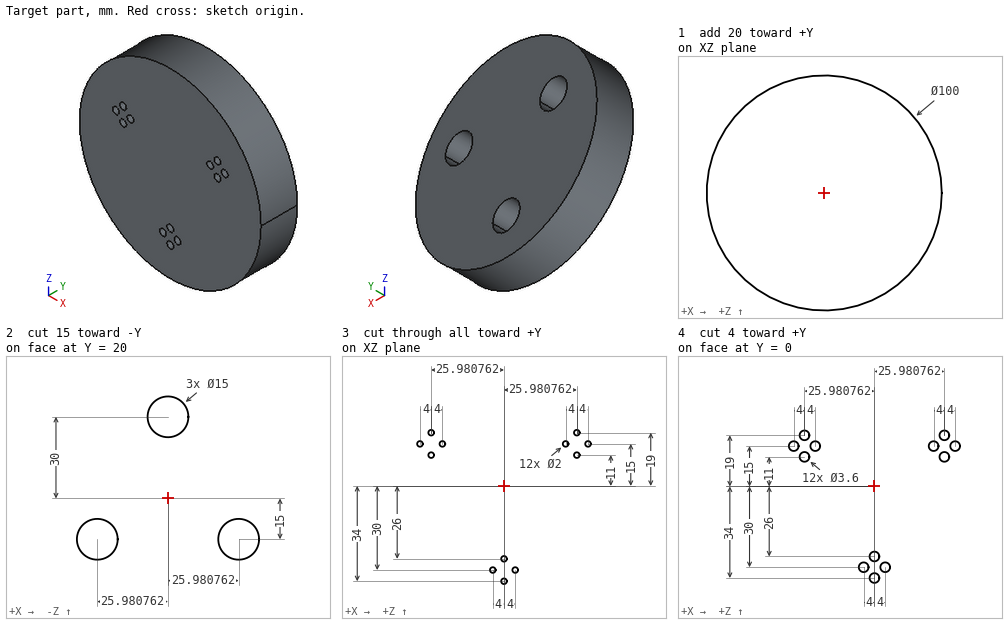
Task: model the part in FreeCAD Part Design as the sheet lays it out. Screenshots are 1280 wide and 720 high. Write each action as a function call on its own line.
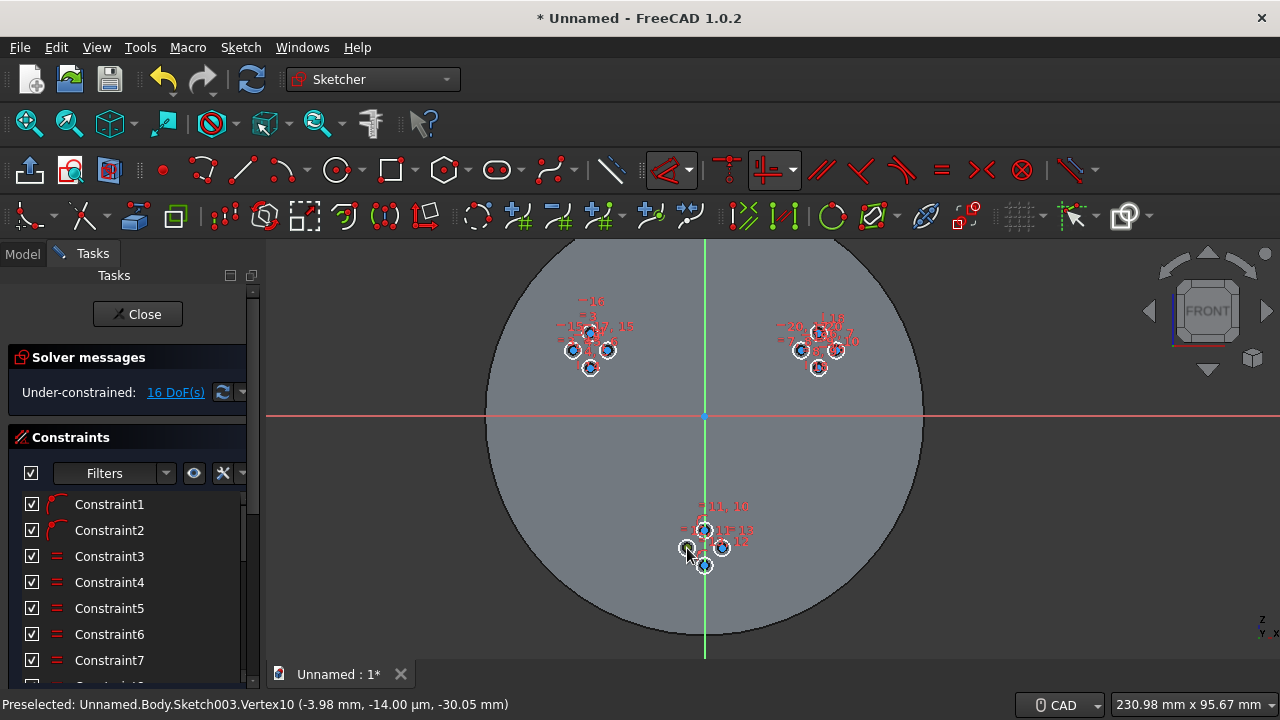
click(722, 548)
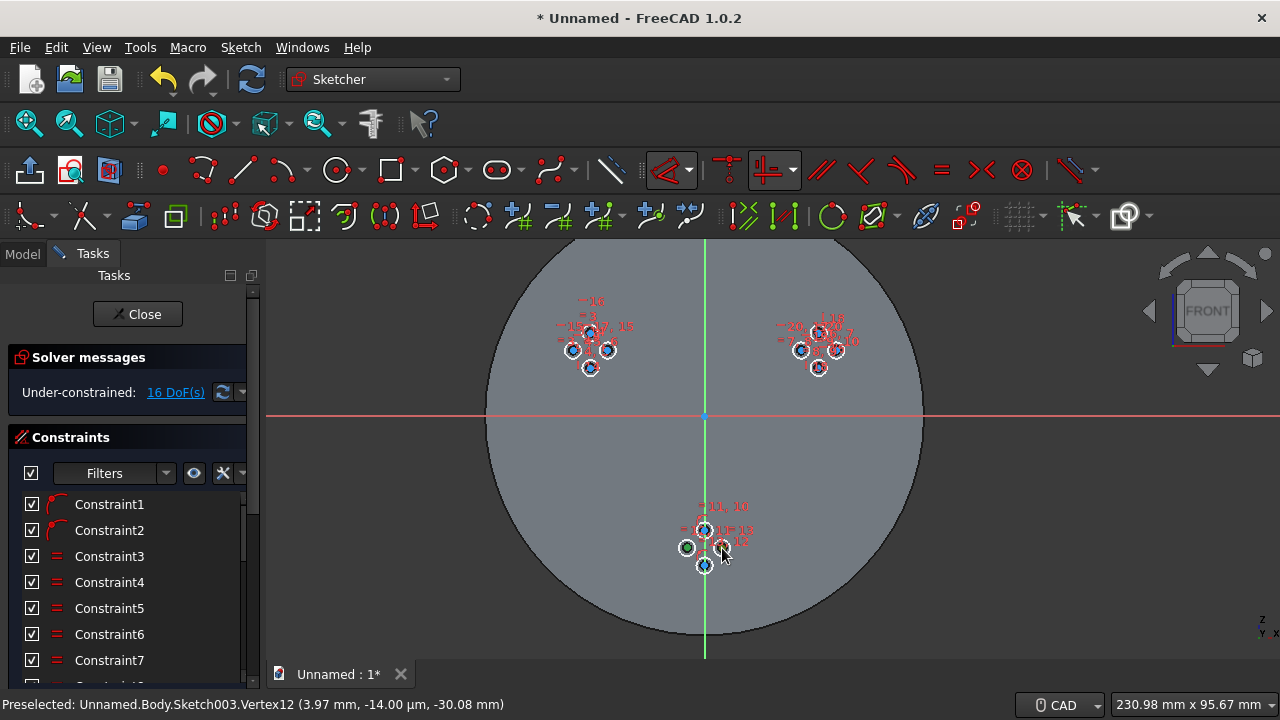
click(796, 170)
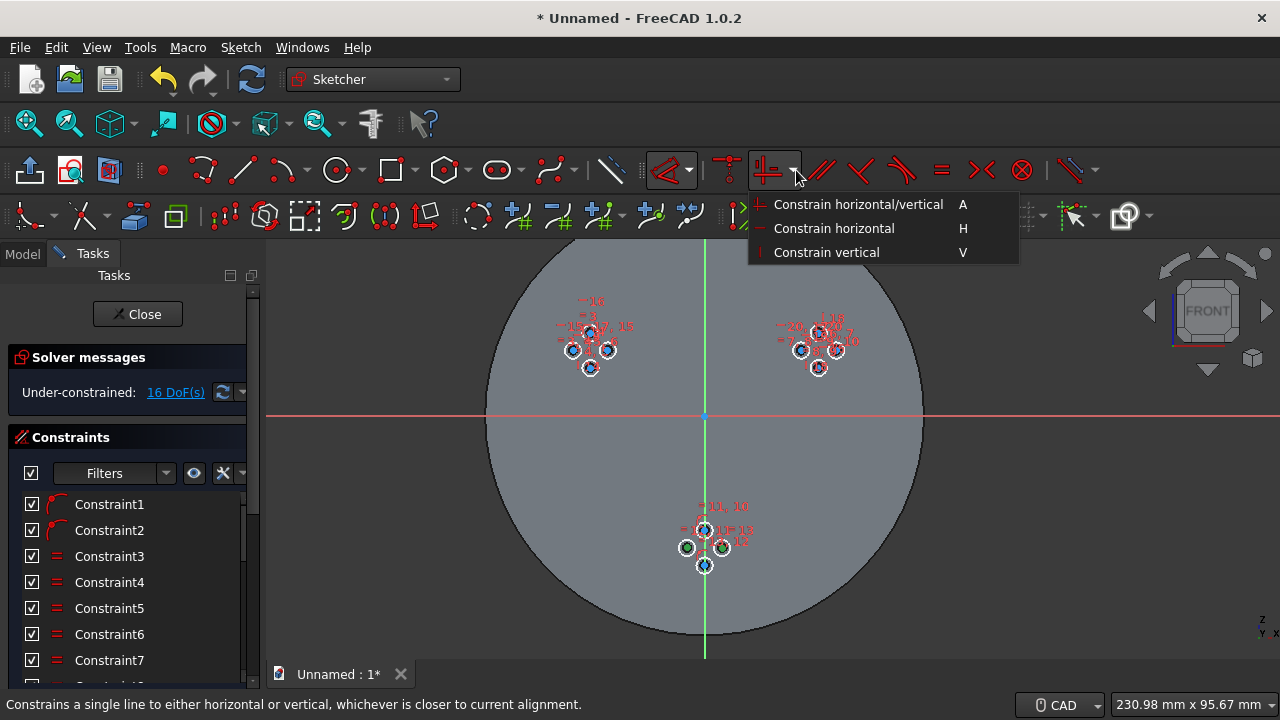
click(884, 228)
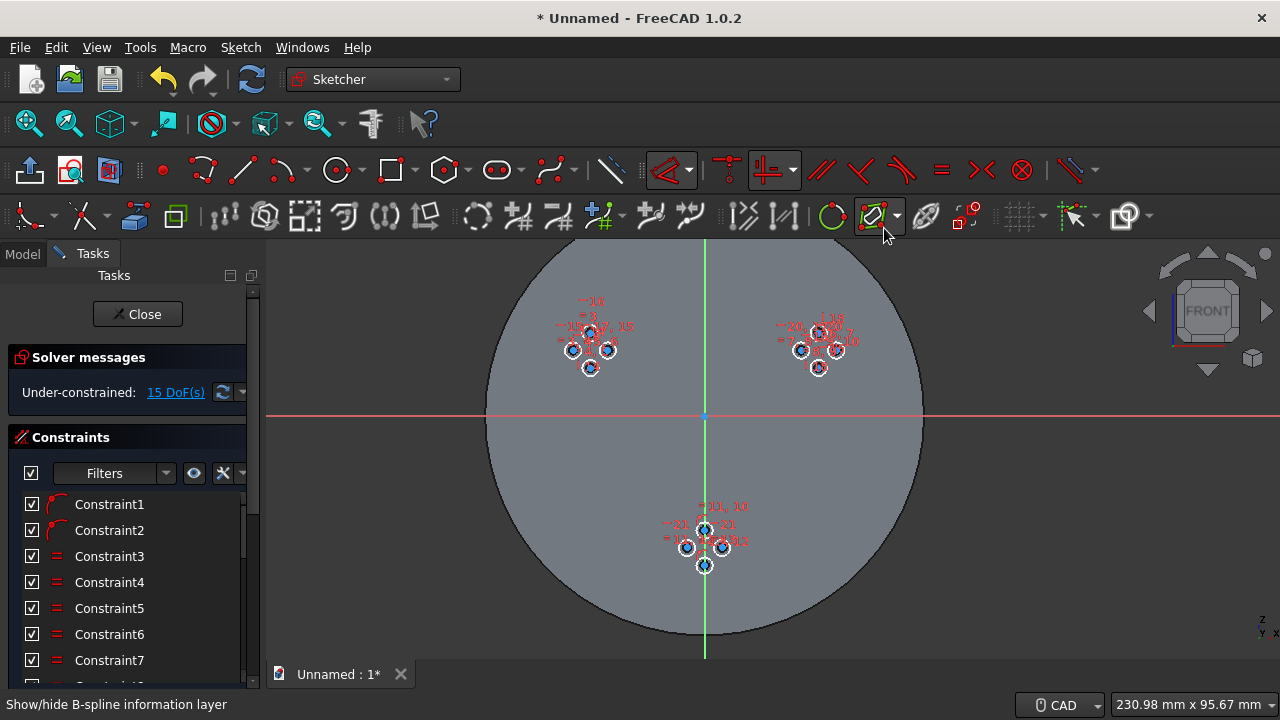
scroll(596, 327, up, 5)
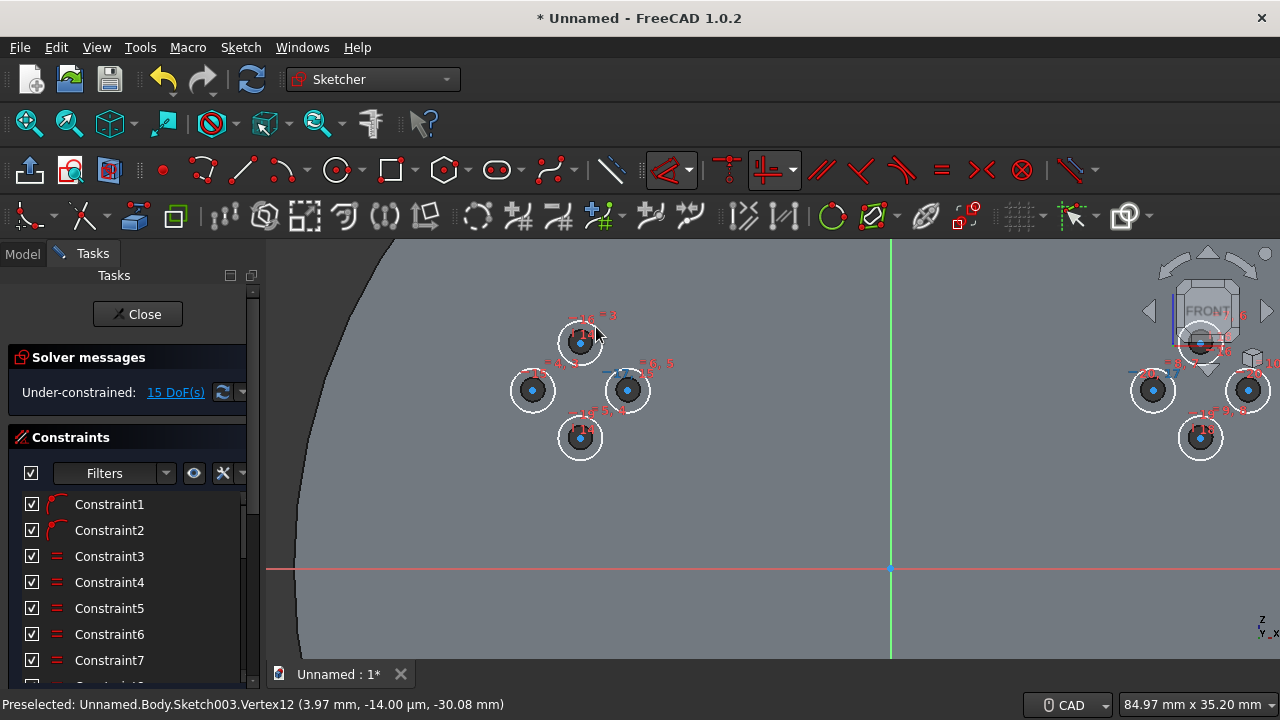
click(596, 328)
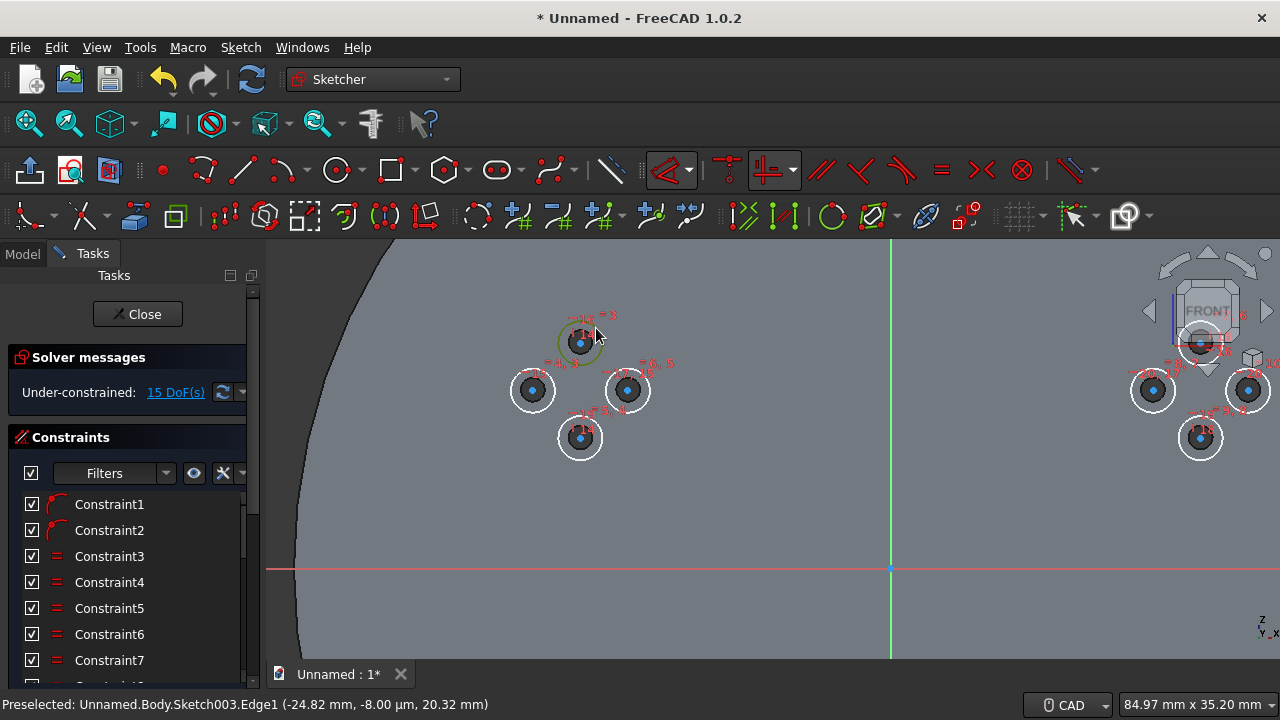
click(692, 170)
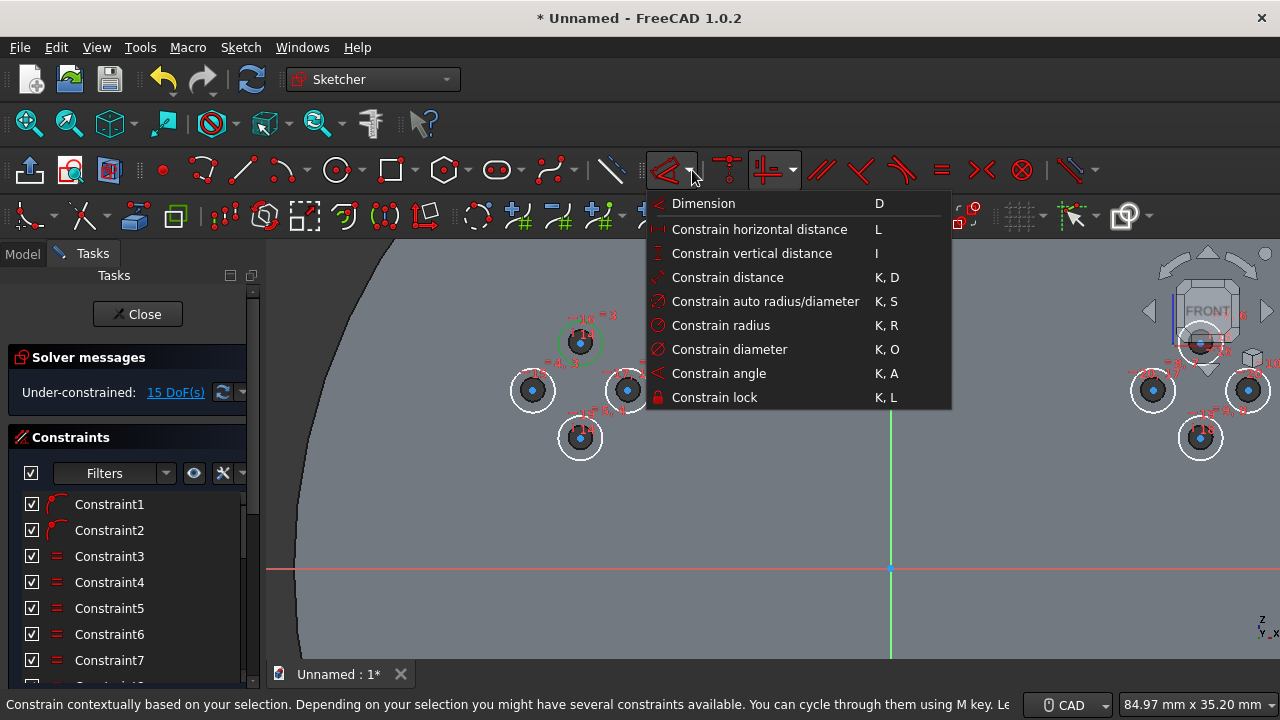
click(799, 349)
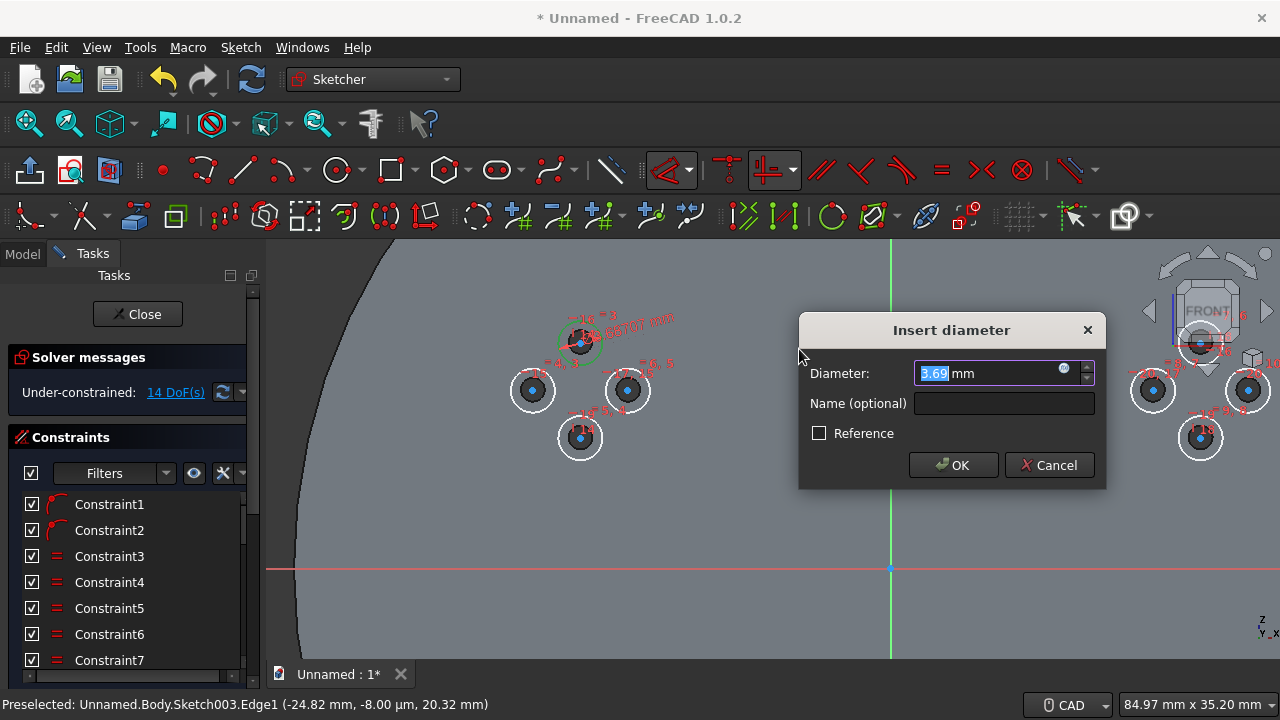
text(3.6)
key(Return)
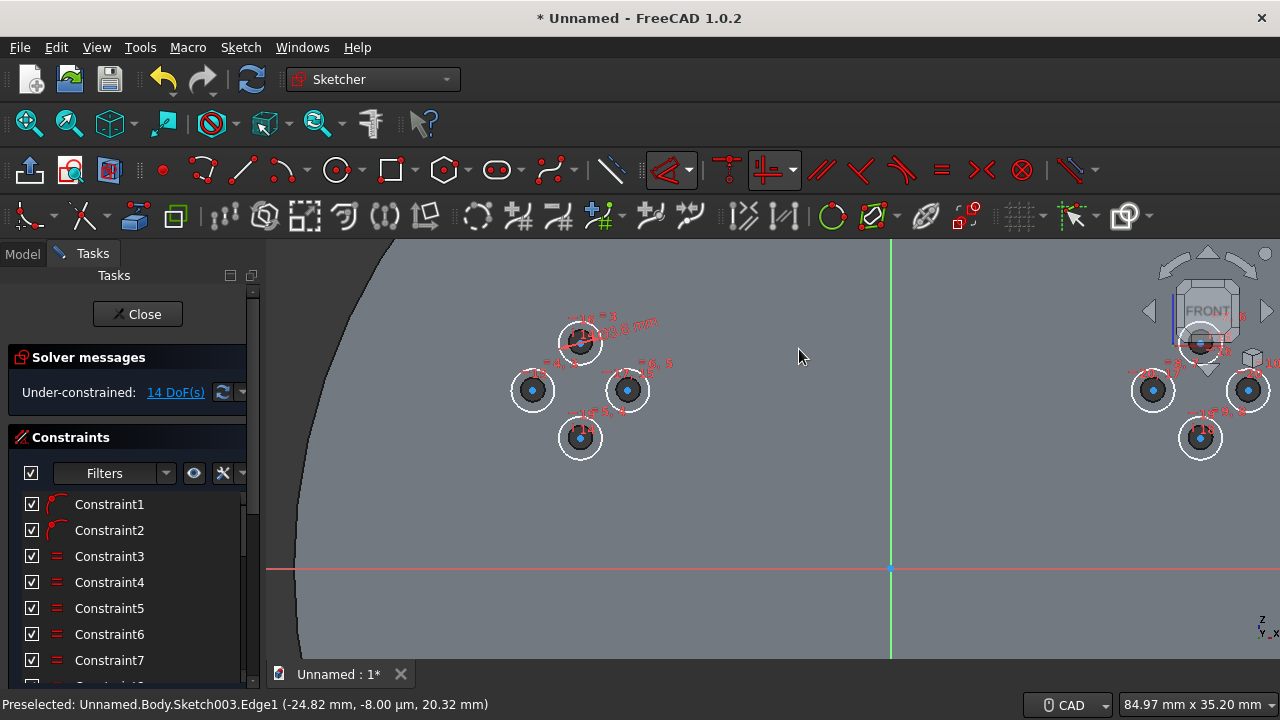
scroll(596, 327, down, 5)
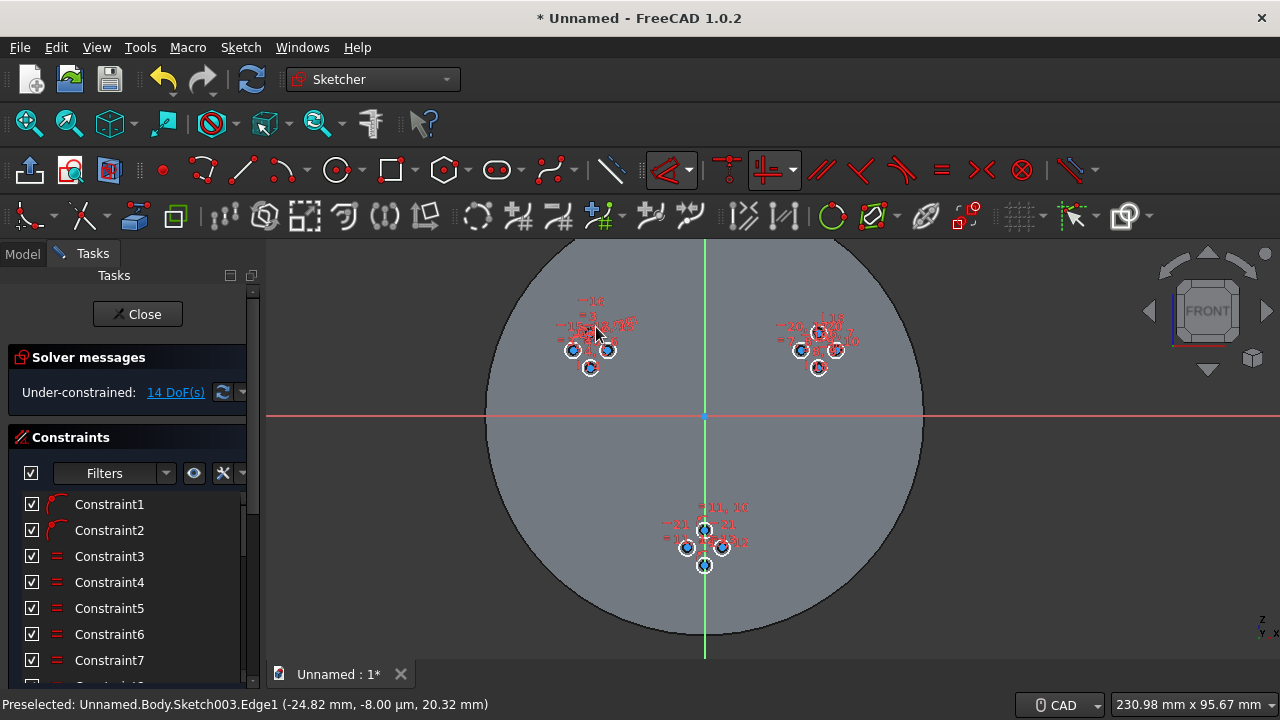
scroll(687, 548, up, 5)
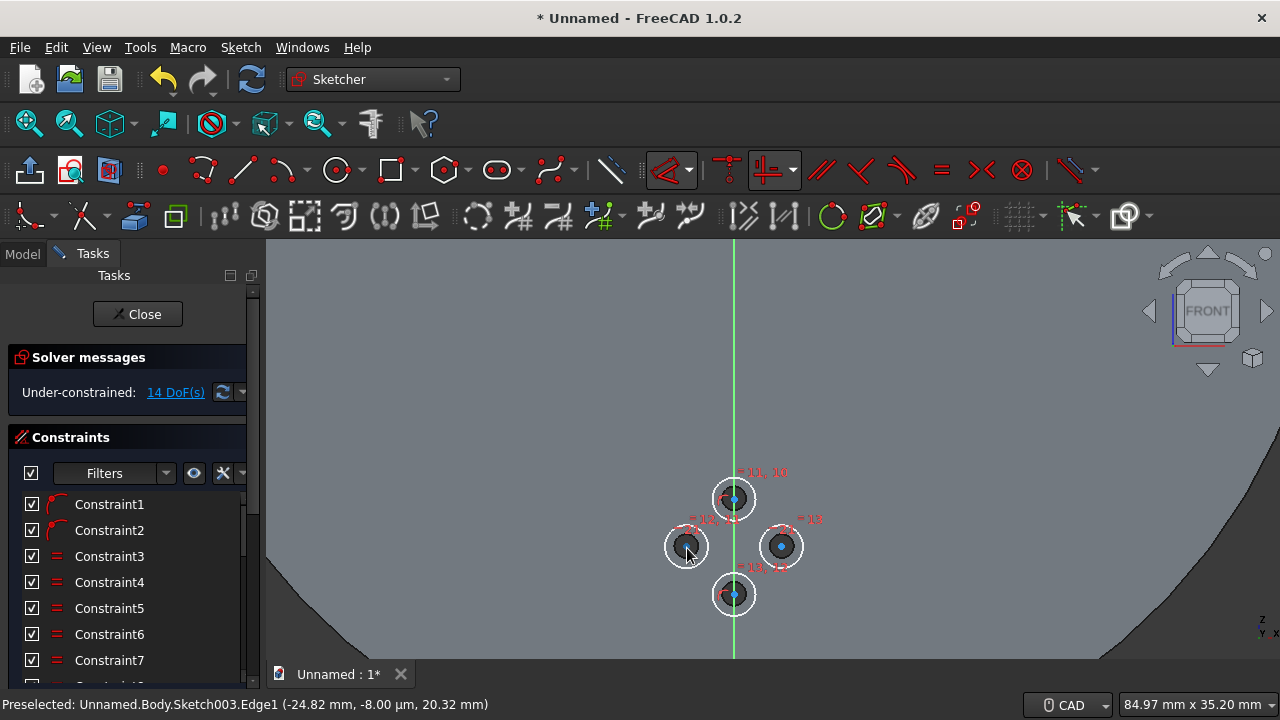
click(687, 547)